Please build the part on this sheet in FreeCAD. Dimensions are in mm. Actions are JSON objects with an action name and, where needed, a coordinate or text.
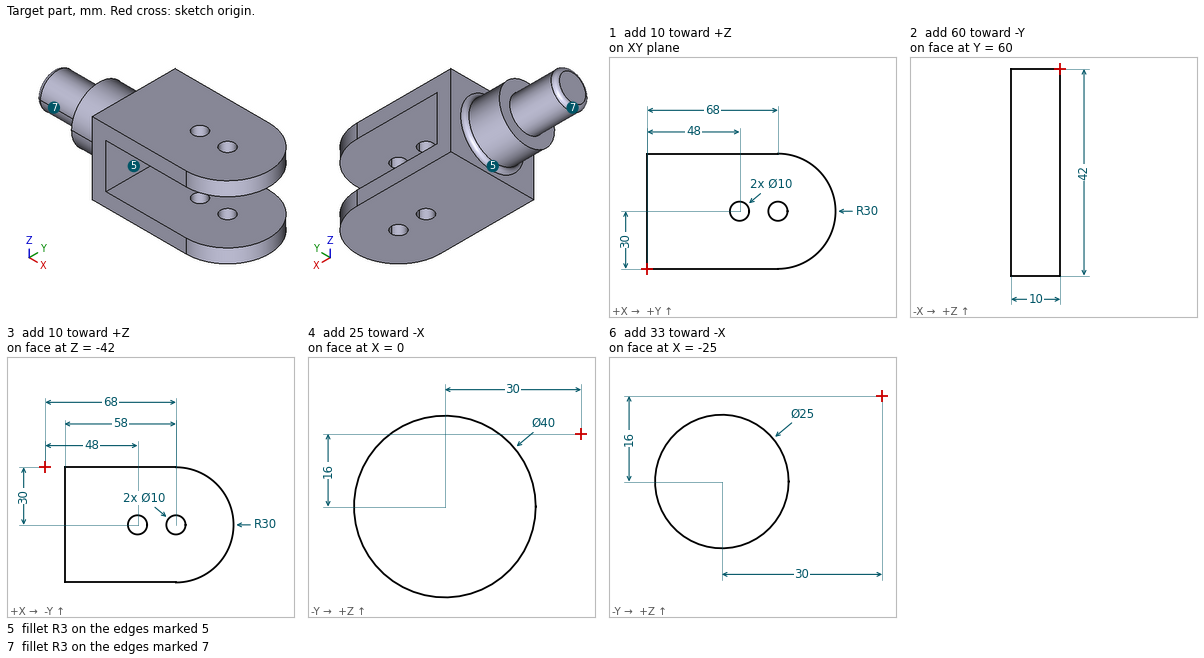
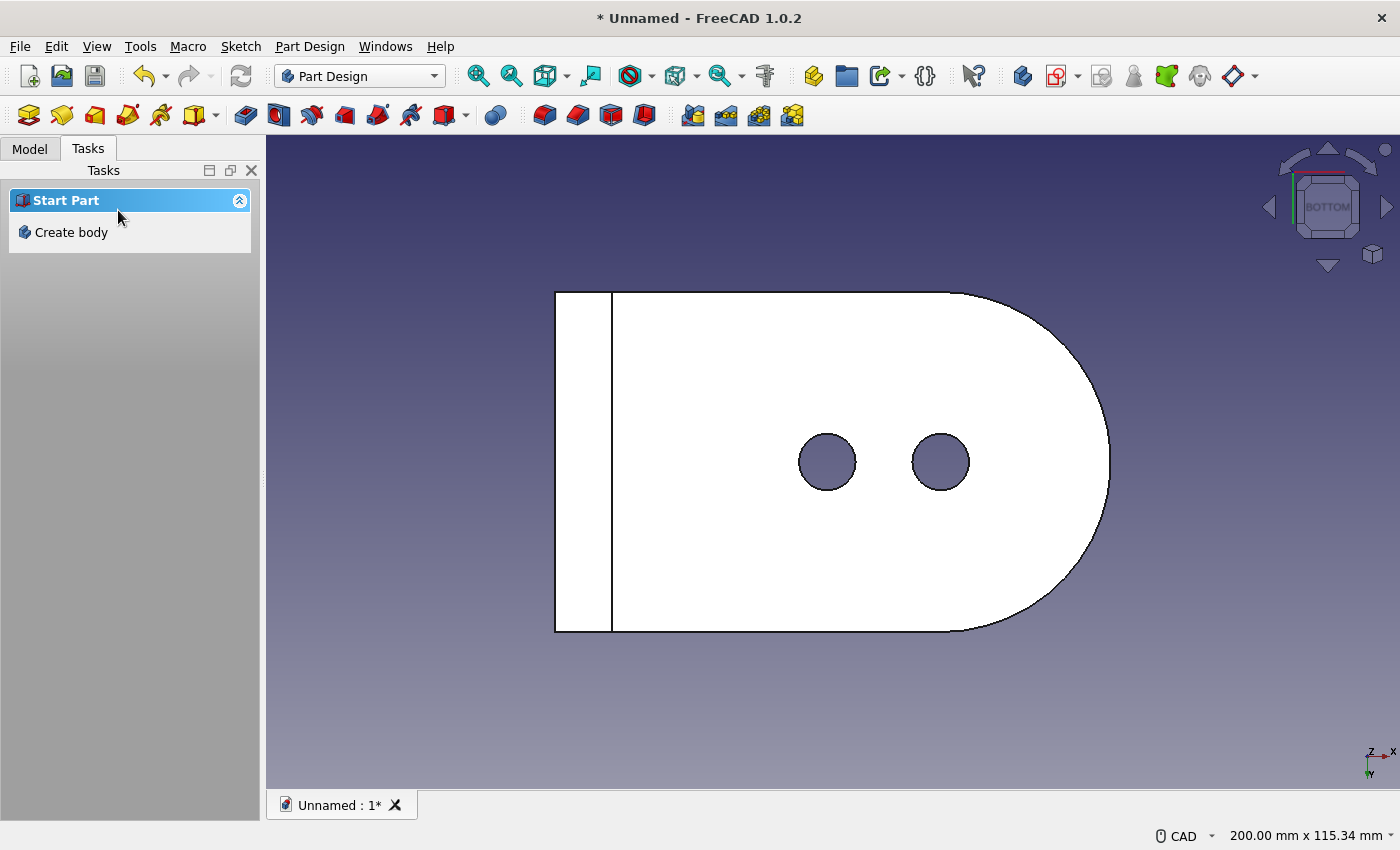
{"action": "left_click", "coordinate": [584, 558]}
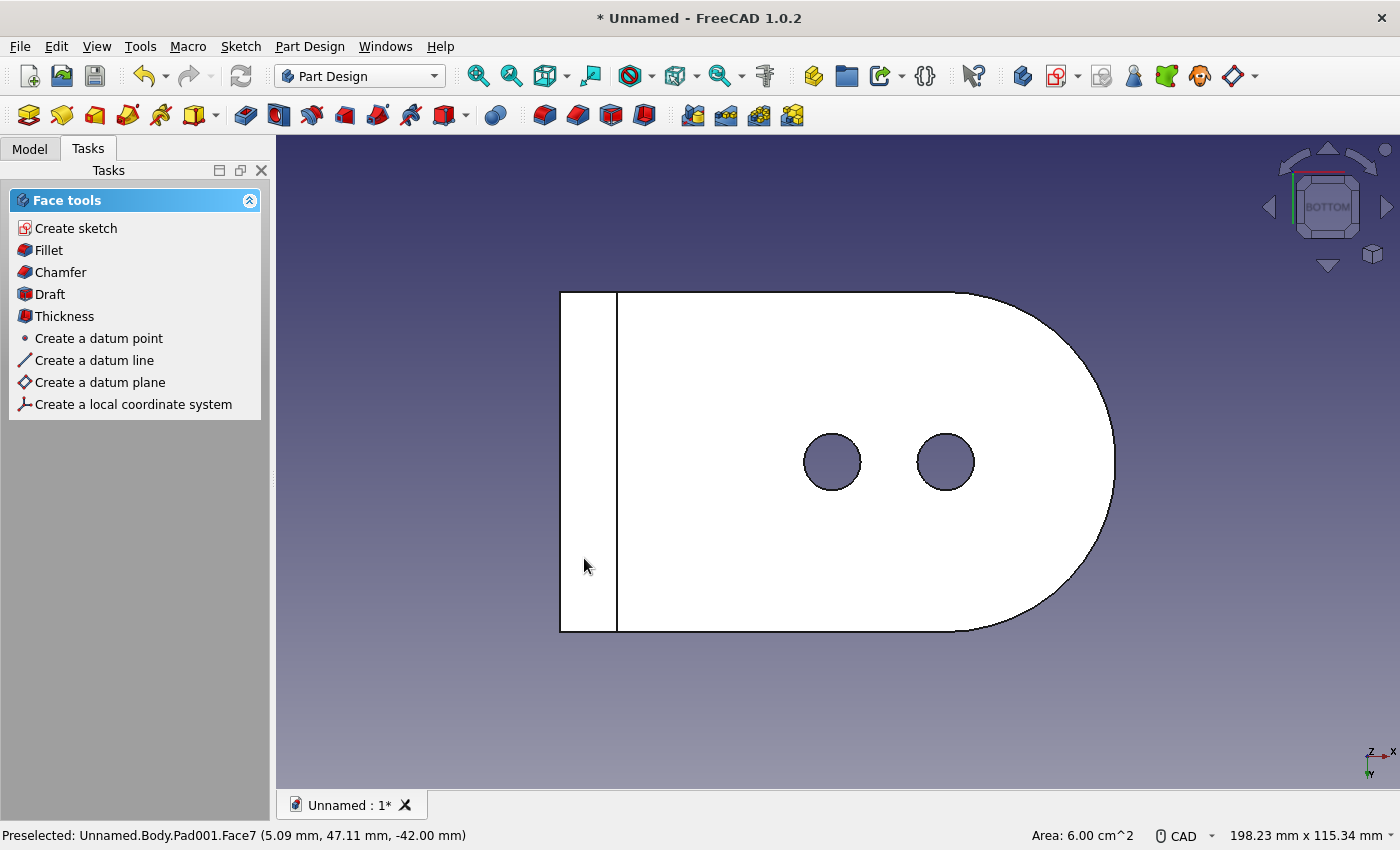
{"action": "left_click", "coordinate": [1056, 76]}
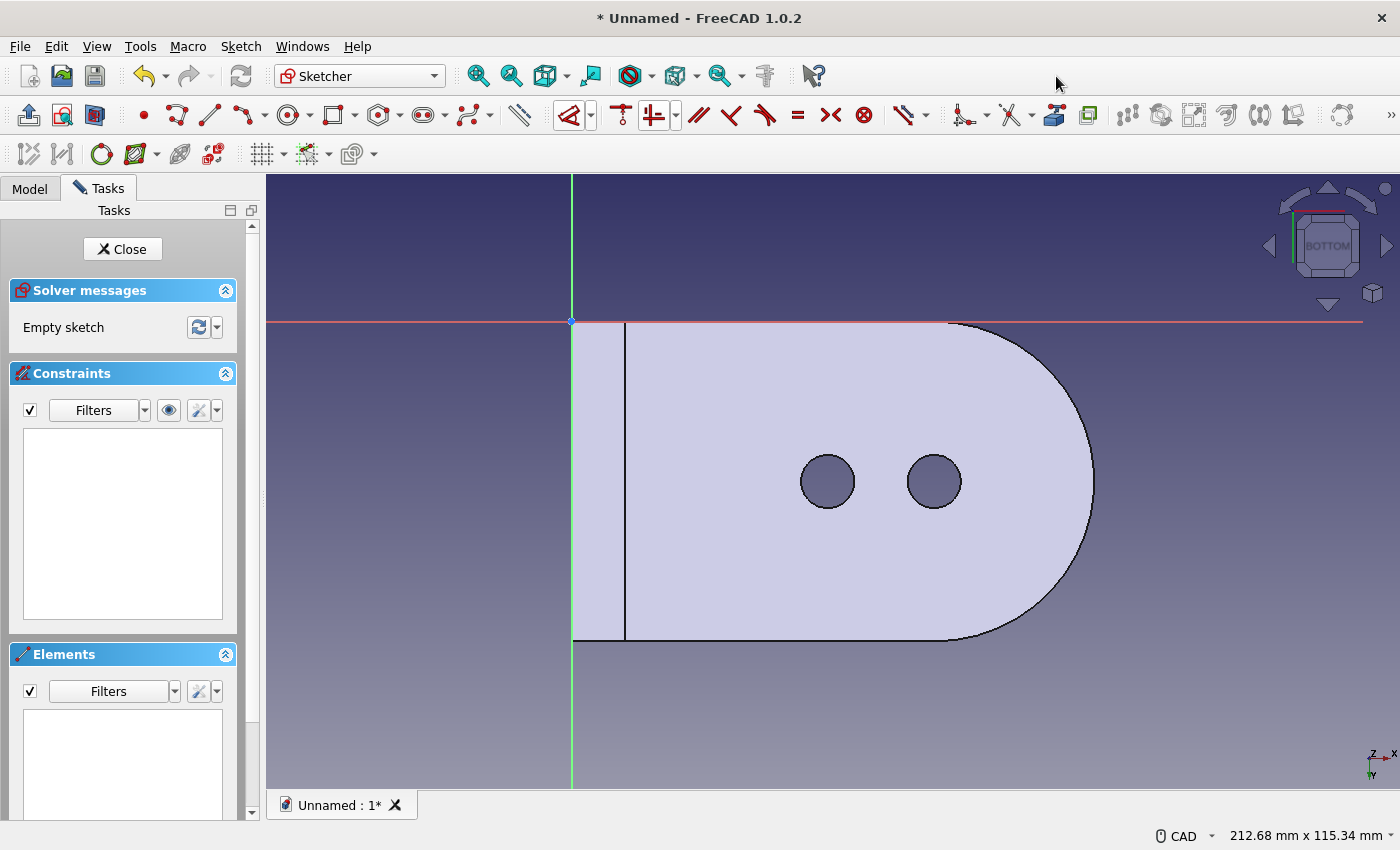
{"action": "key", "text": "g m"}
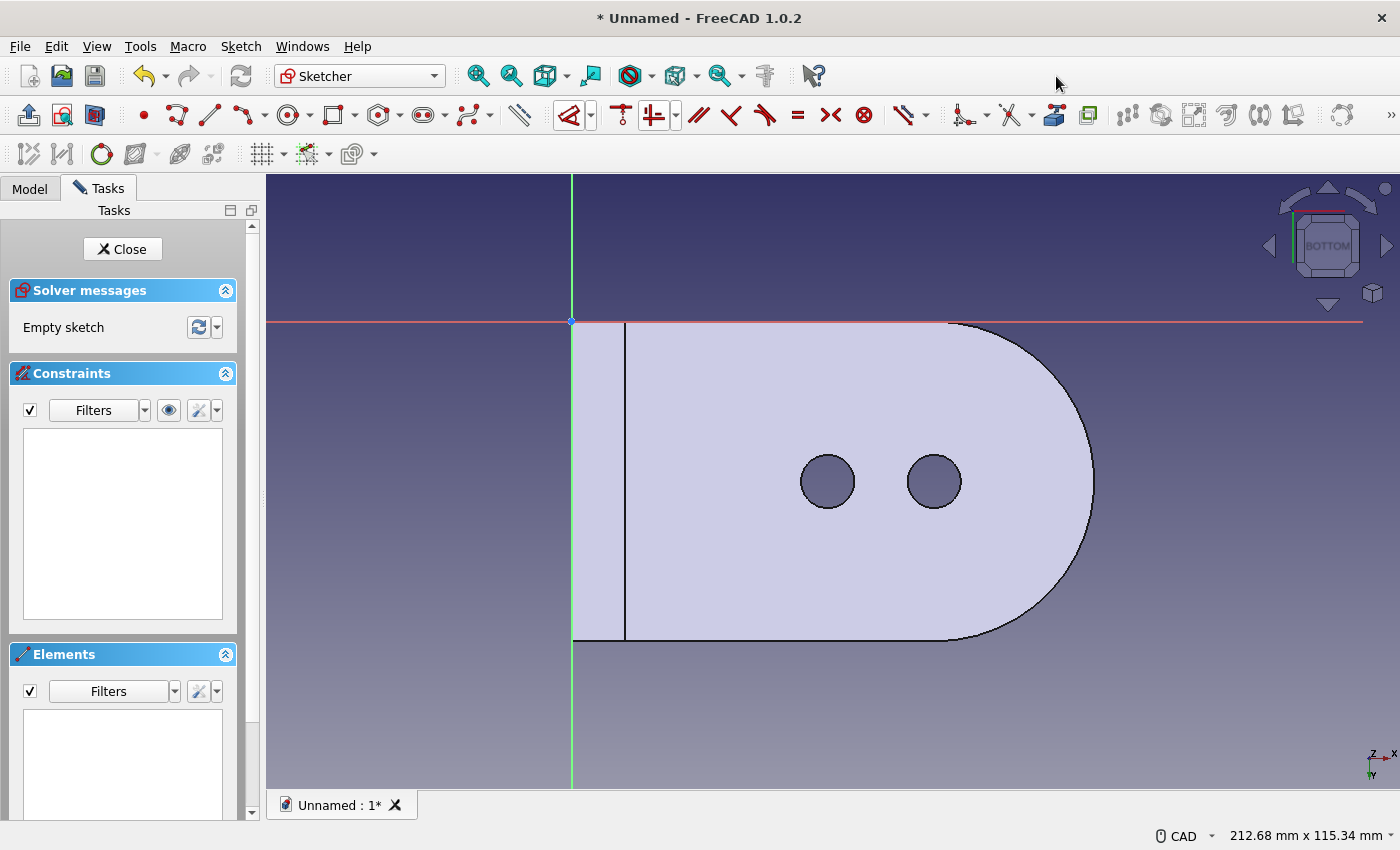
{"action": "left_click", "coordinate": [934, 322]}
{"action": "left_click", "coordinate": [625, 331]}
{"action": "left_click", "coordinate": [625, 641]}
{"action": "left_click", "coordinate": [934, 641]}
{"action": "right_click", "coordinate": [934, 641]}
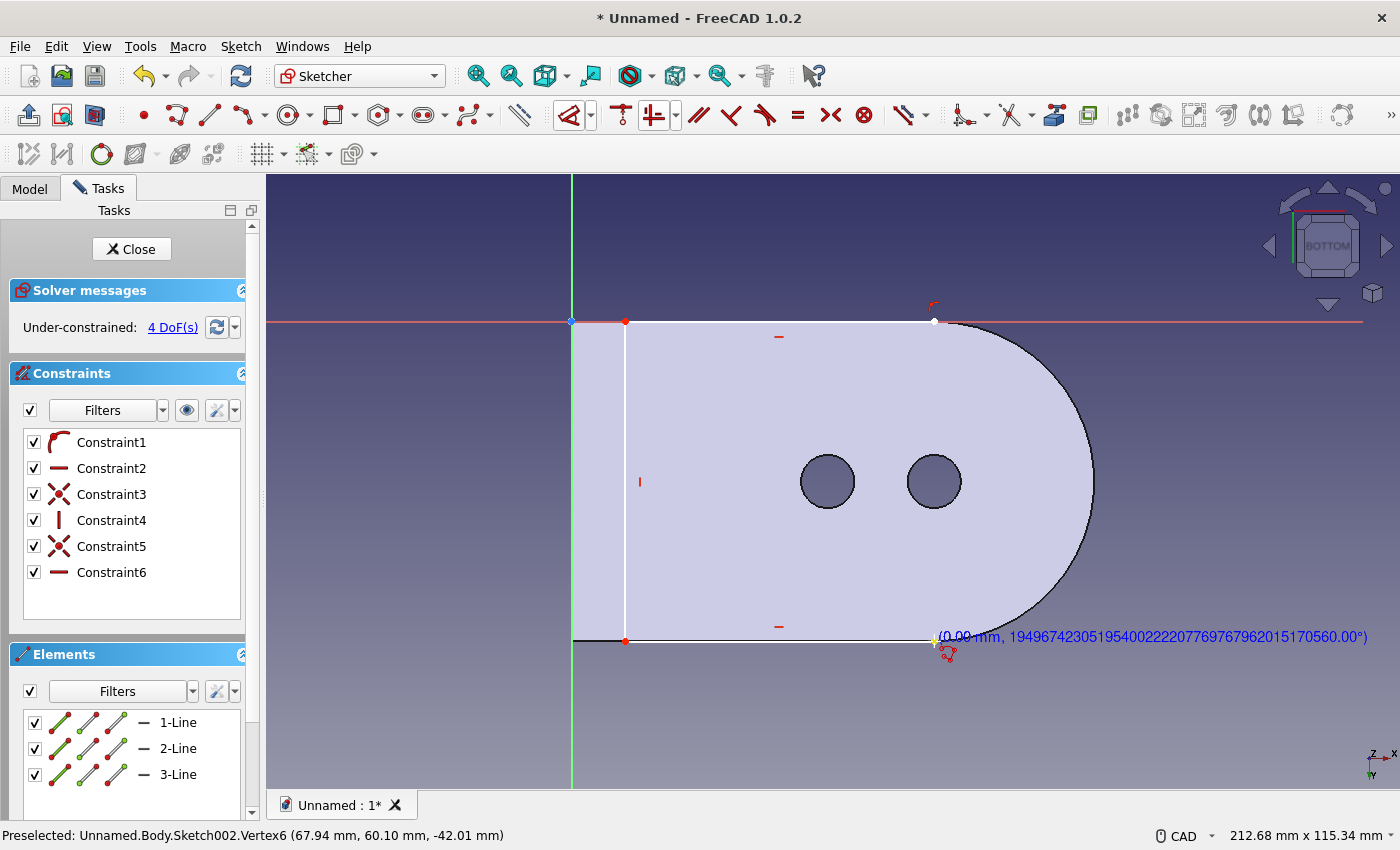
{"action": "key", "text": "g 3 a"}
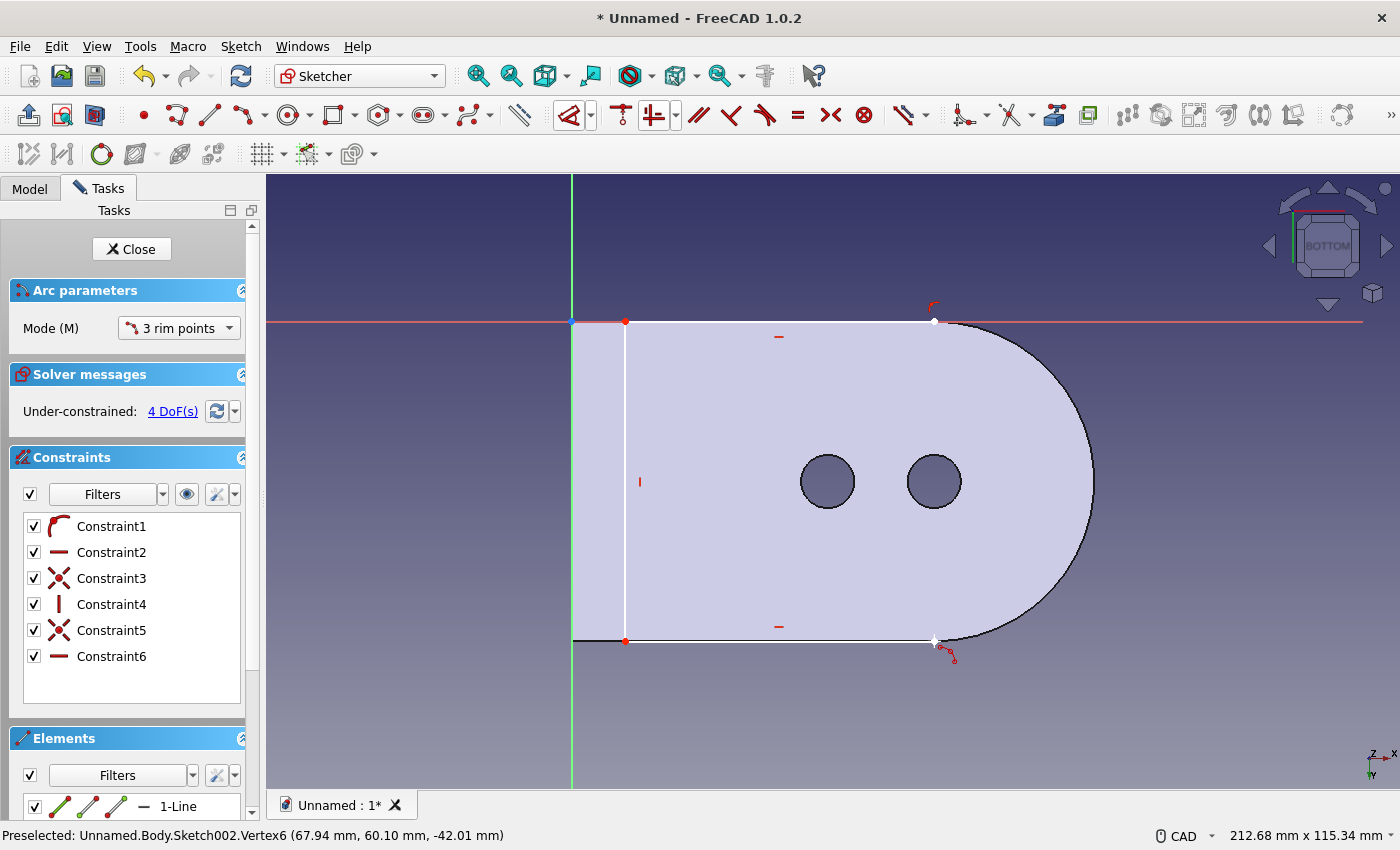
{"action": "left_click", "coordinate": [934, 642]}
{"action": "left_click", "coordinate": [934, 322]}
{"action": "left_click", "coordinate": [1094, 482]}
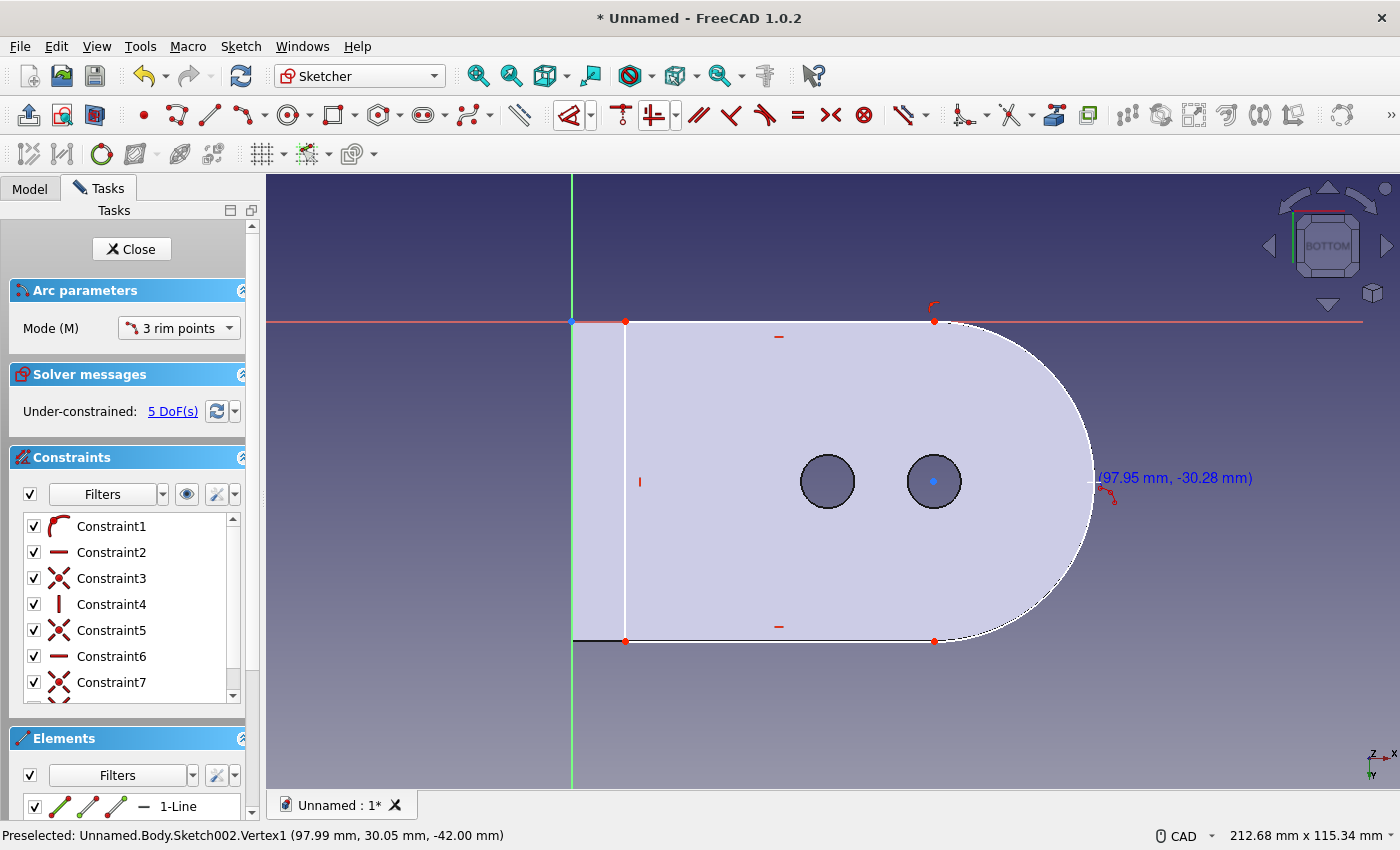
{"action": "key", "text": "g c"}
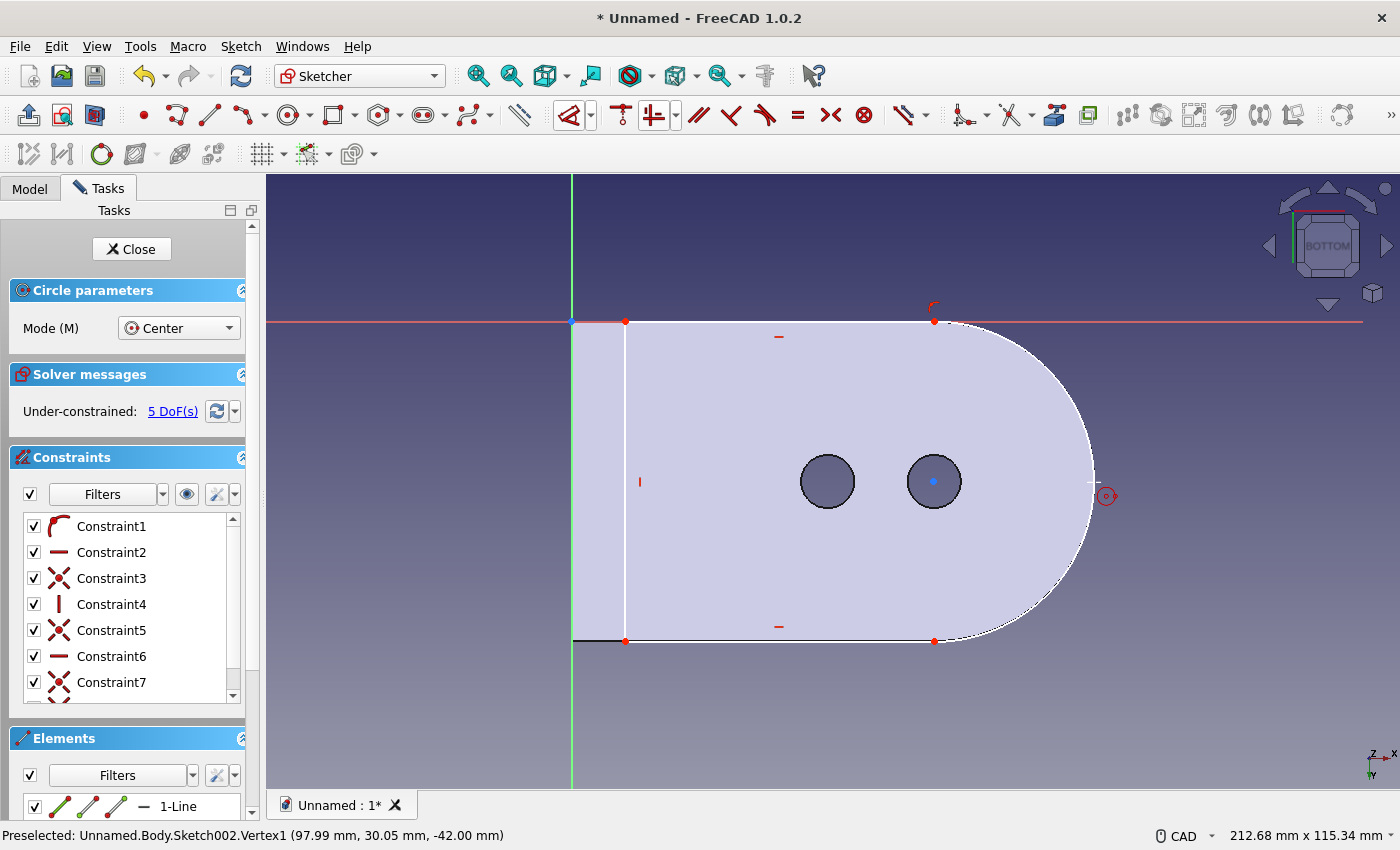
{"action": "left_click", "coordinate": [934, 482]}
{"action": "mouse_move", "coordinate": [953, 463]}